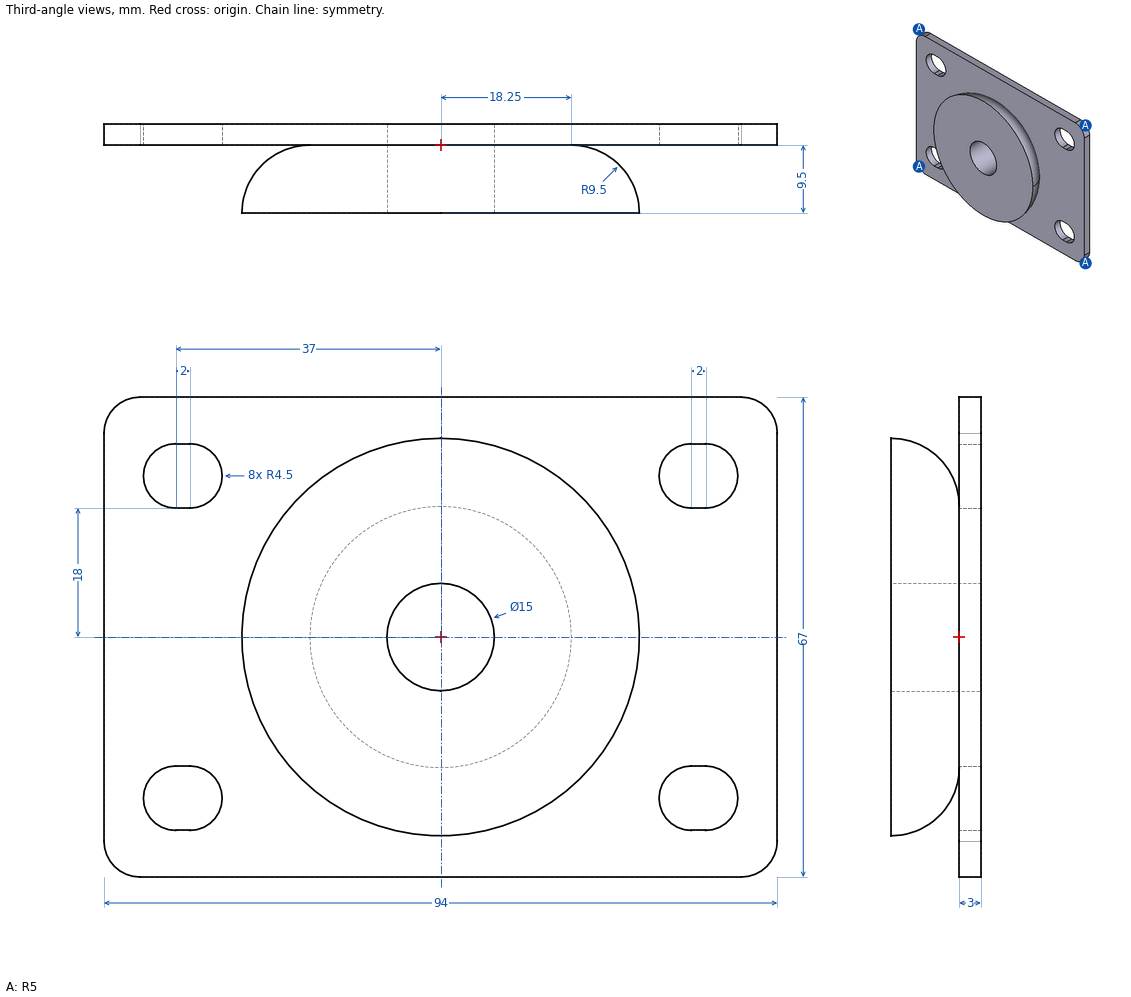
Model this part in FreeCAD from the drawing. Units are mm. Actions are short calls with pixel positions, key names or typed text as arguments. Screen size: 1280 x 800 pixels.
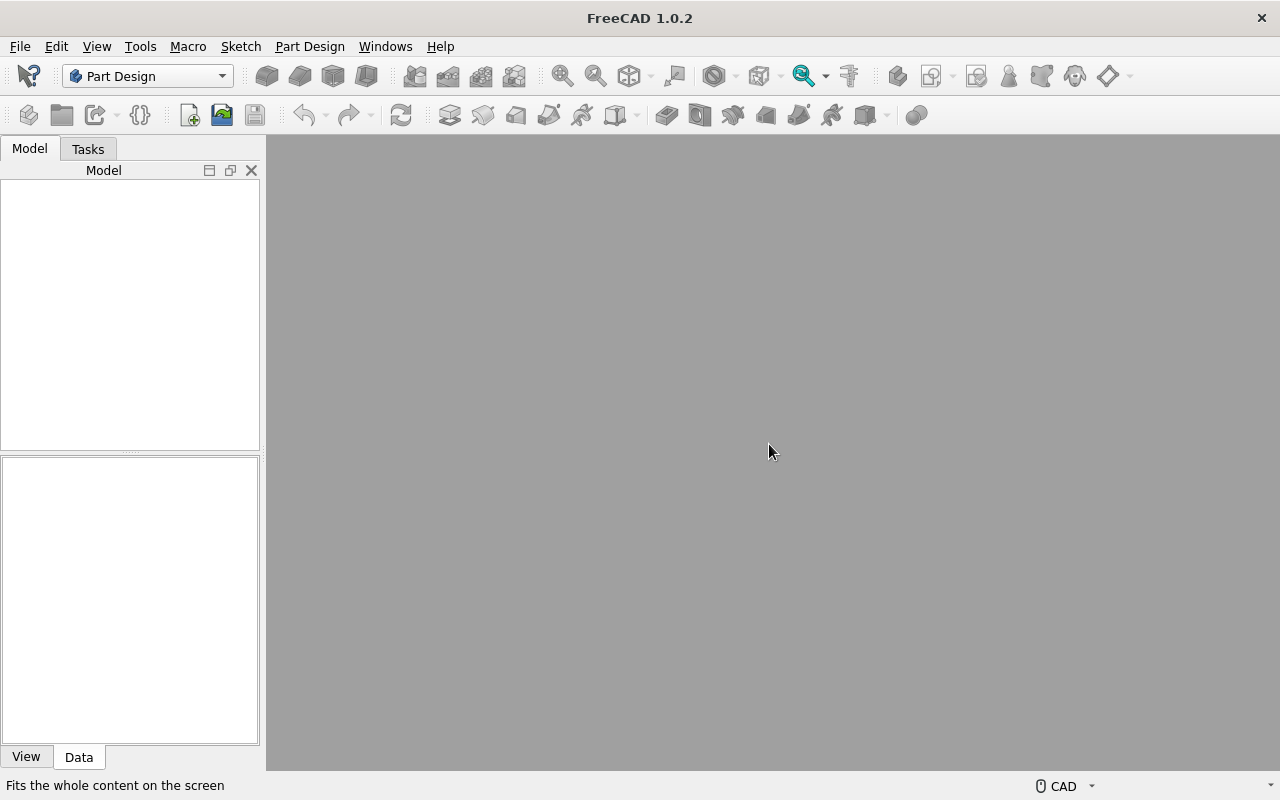
key(ctrl+n)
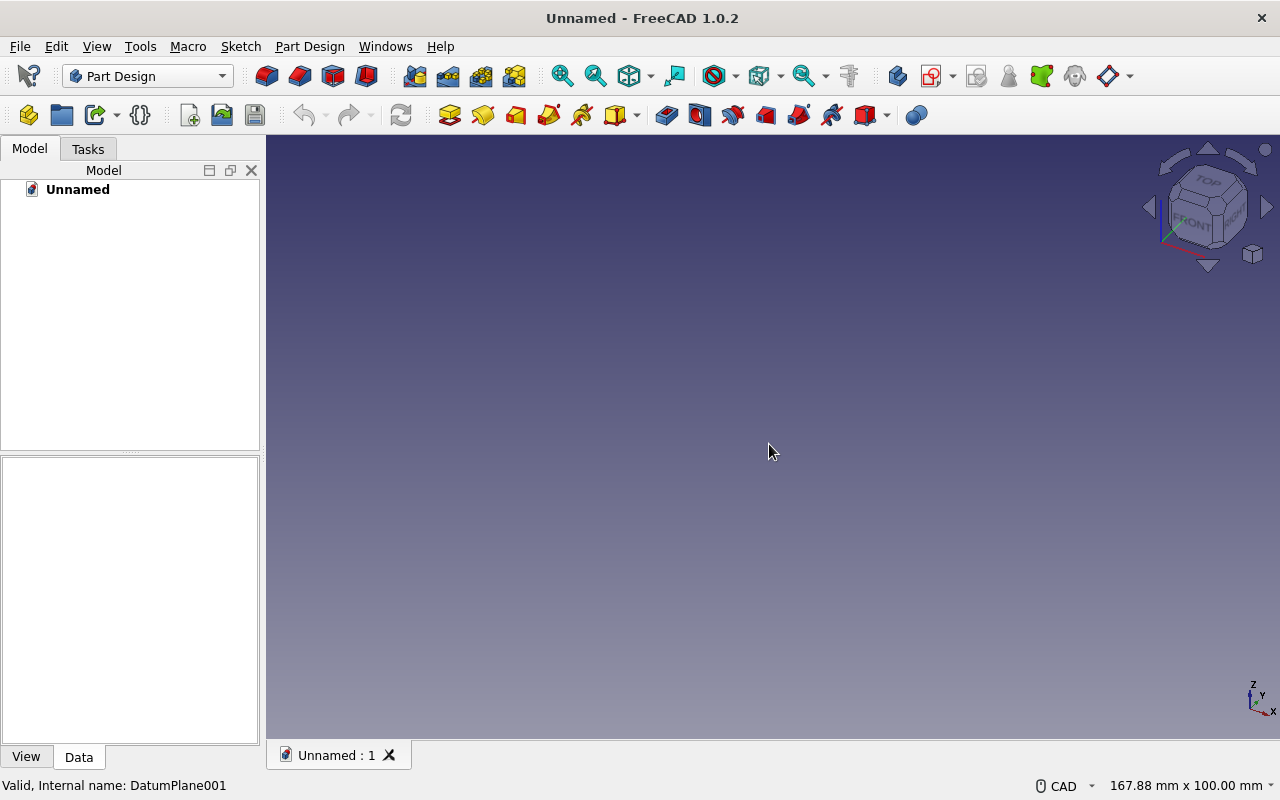
click(930, 76)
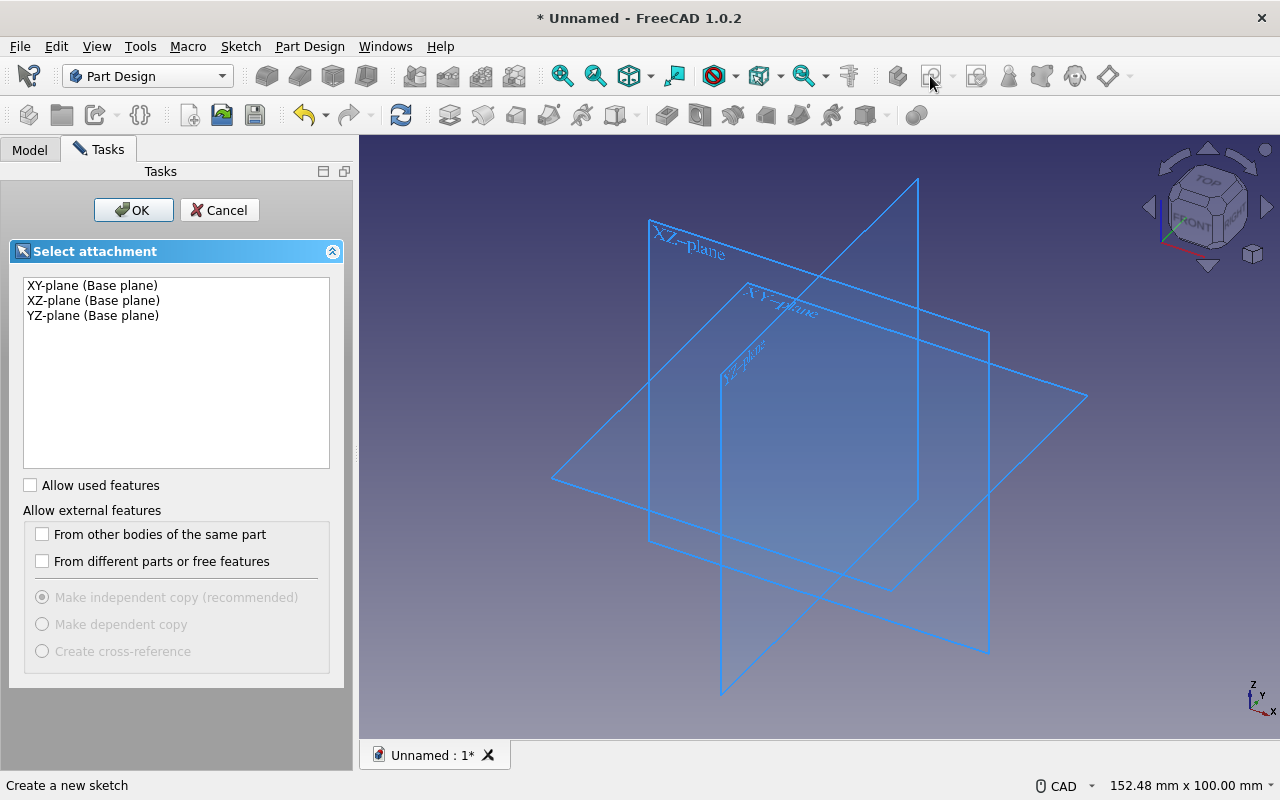
click(84, 300)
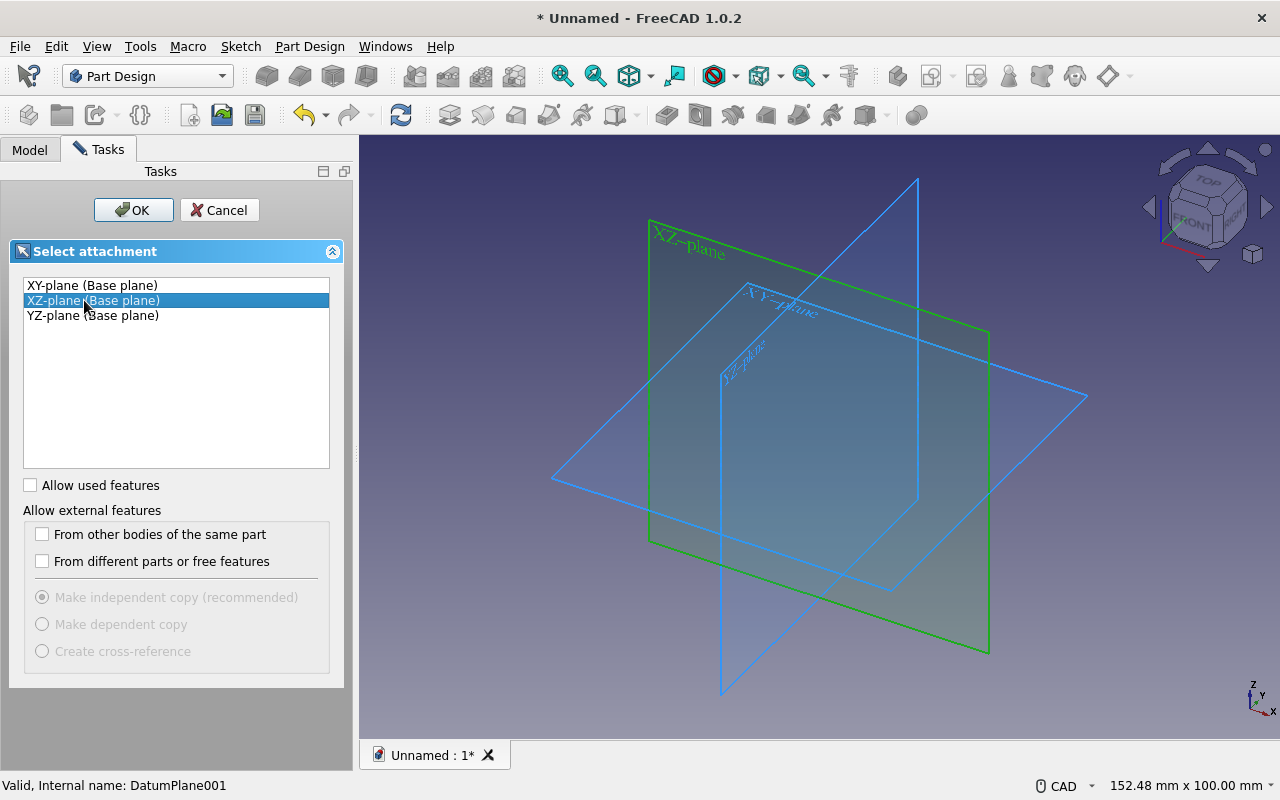
click(134, 210)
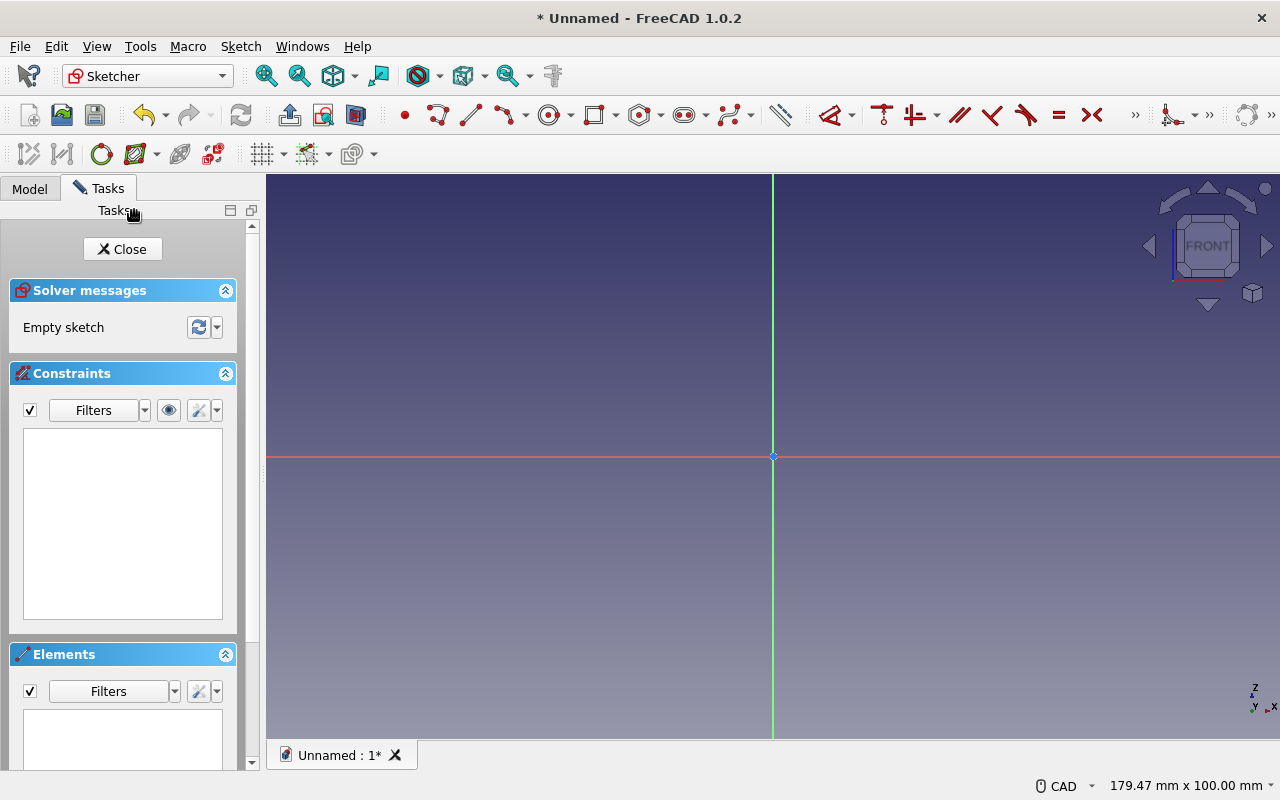
key(g)
key(v)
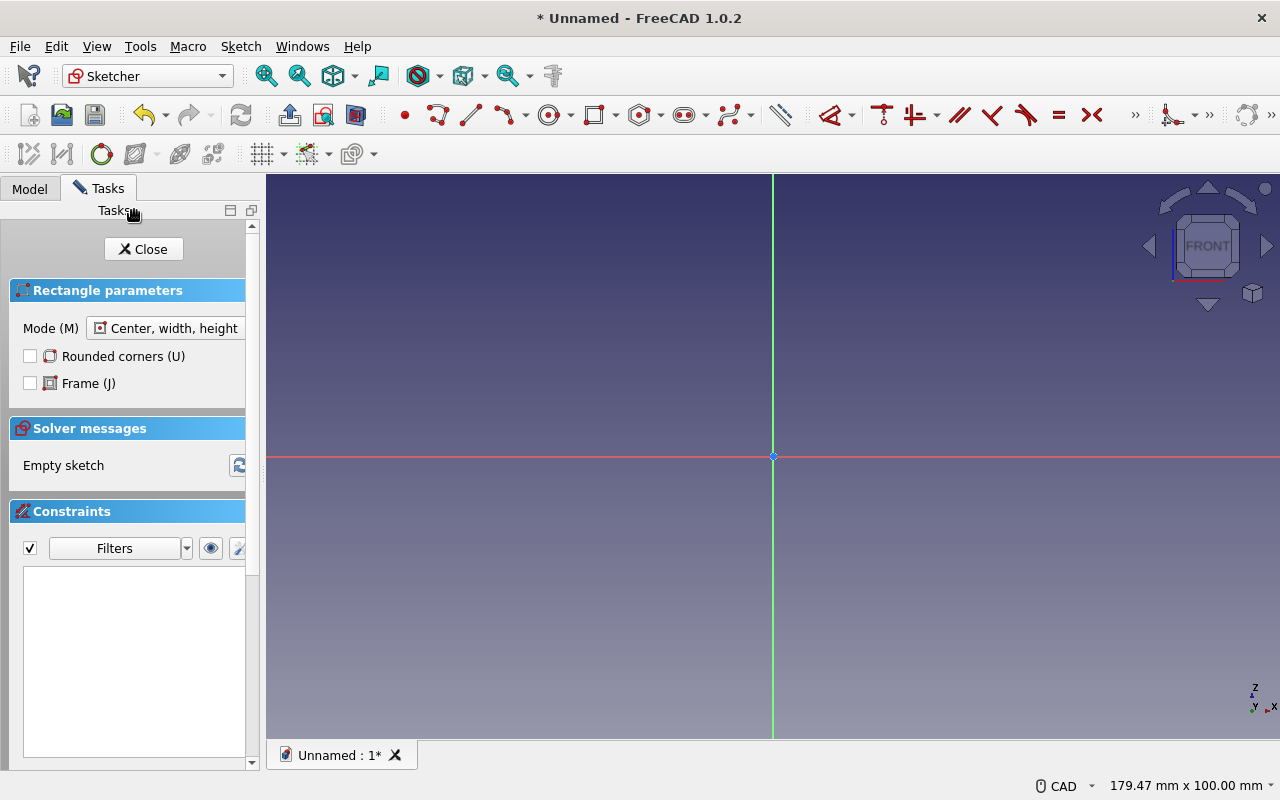
click(773, 456)
move(1039, 267)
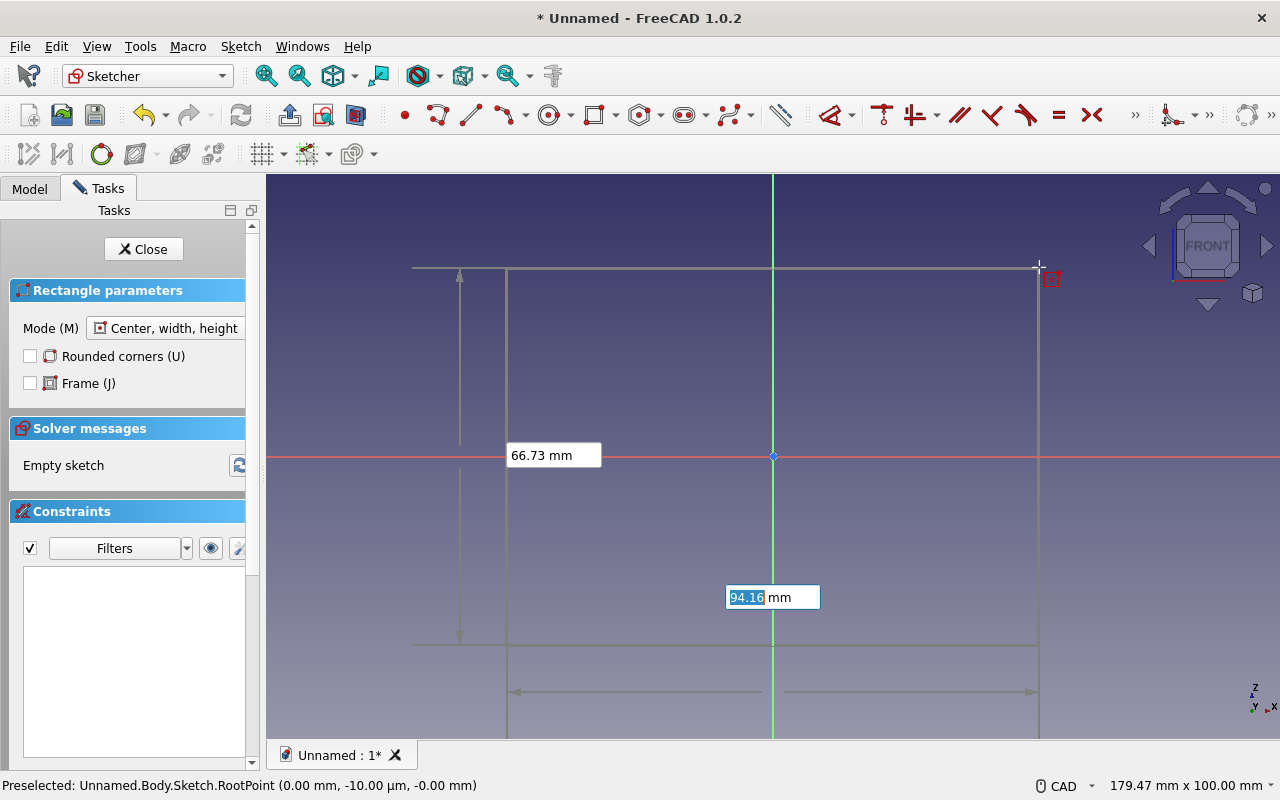
text(94)
key(Tab)
text(67)
key(Return)
key(Escape)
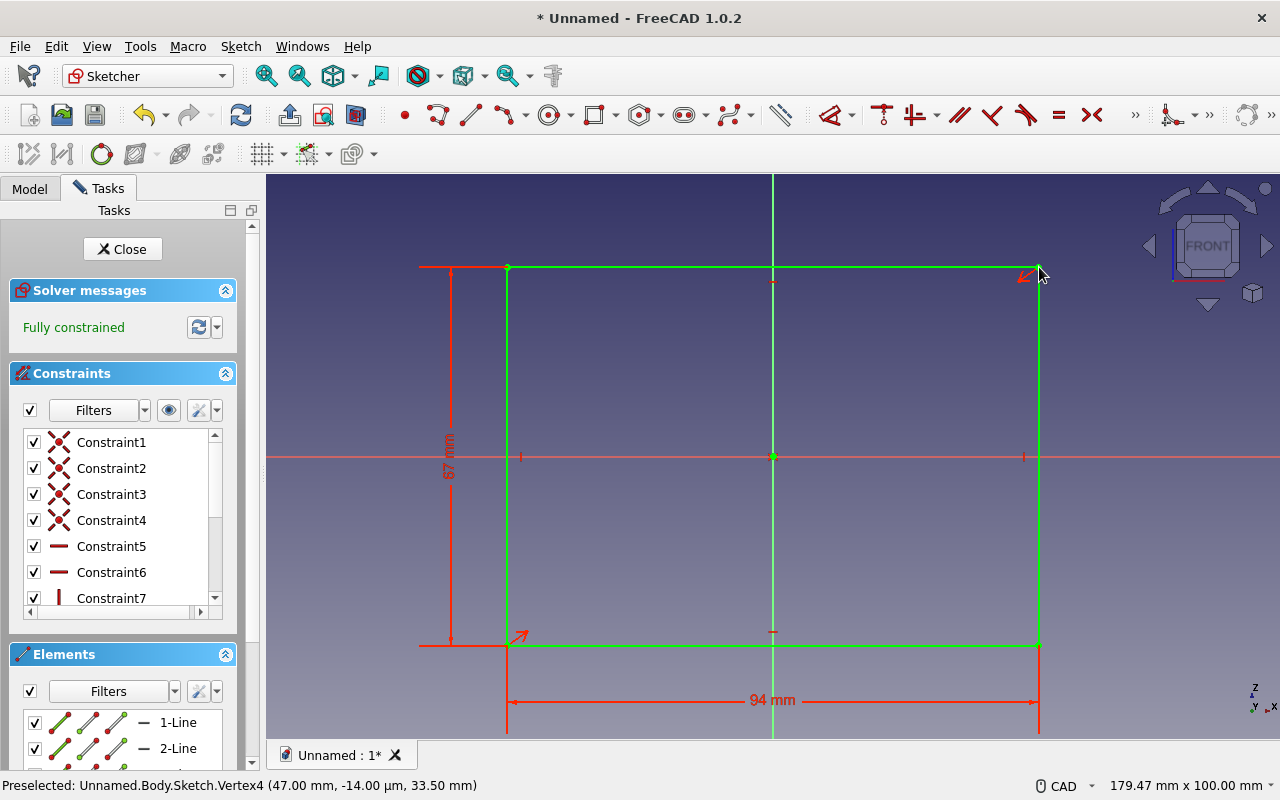
click(123, 249)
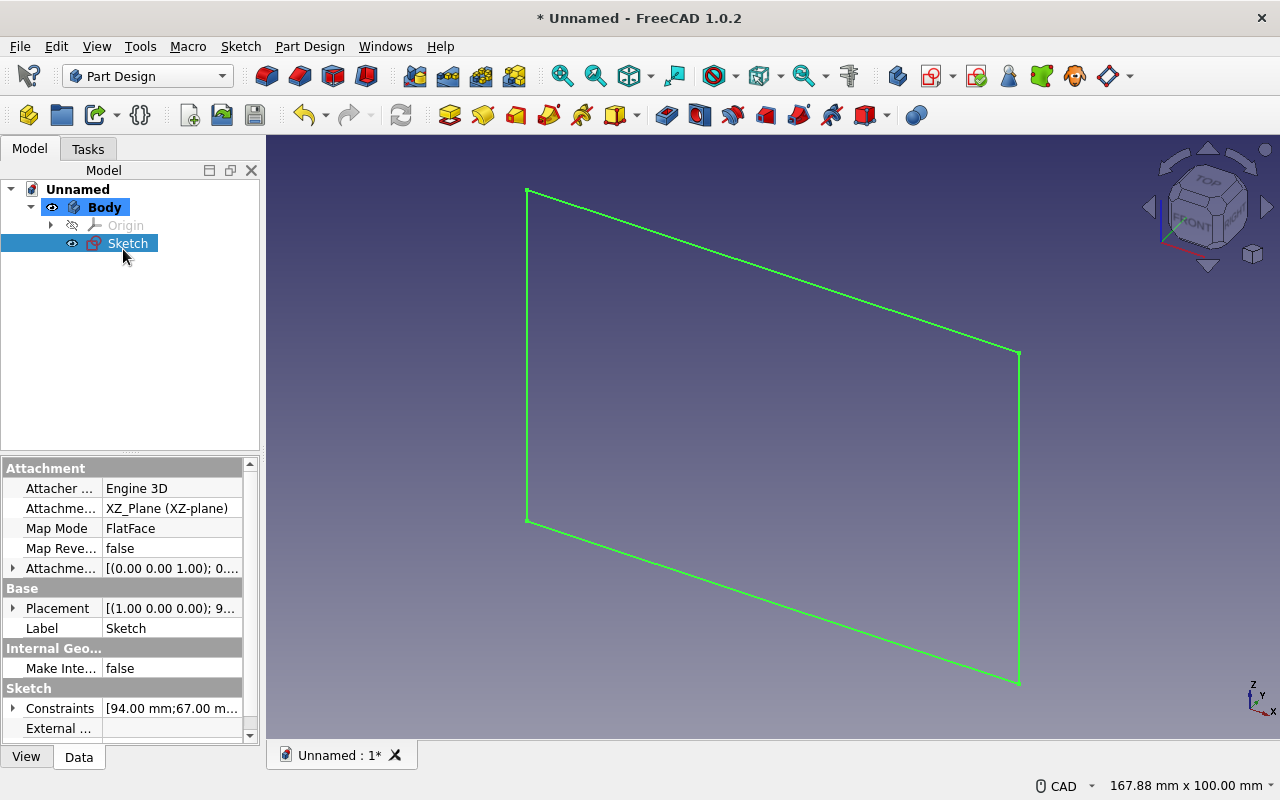
click(450, 116)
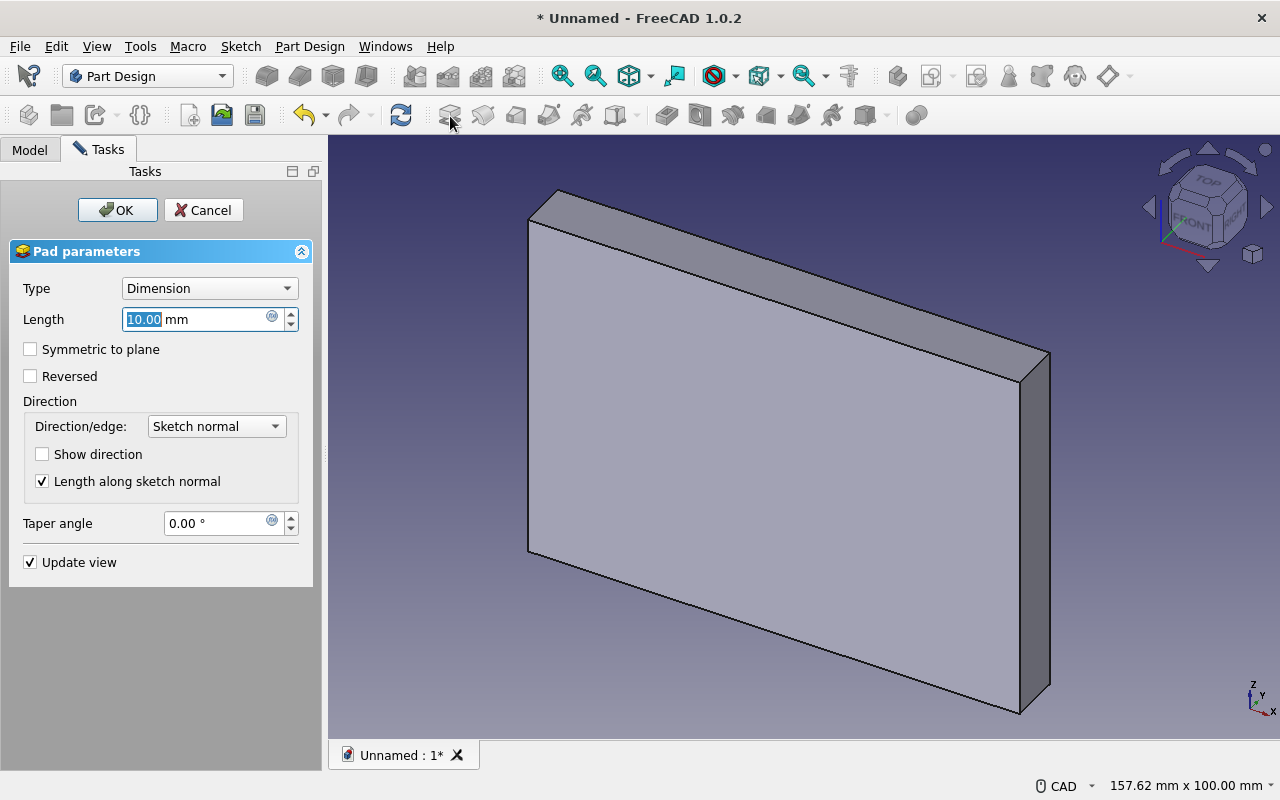
text(3)
key(Tab)